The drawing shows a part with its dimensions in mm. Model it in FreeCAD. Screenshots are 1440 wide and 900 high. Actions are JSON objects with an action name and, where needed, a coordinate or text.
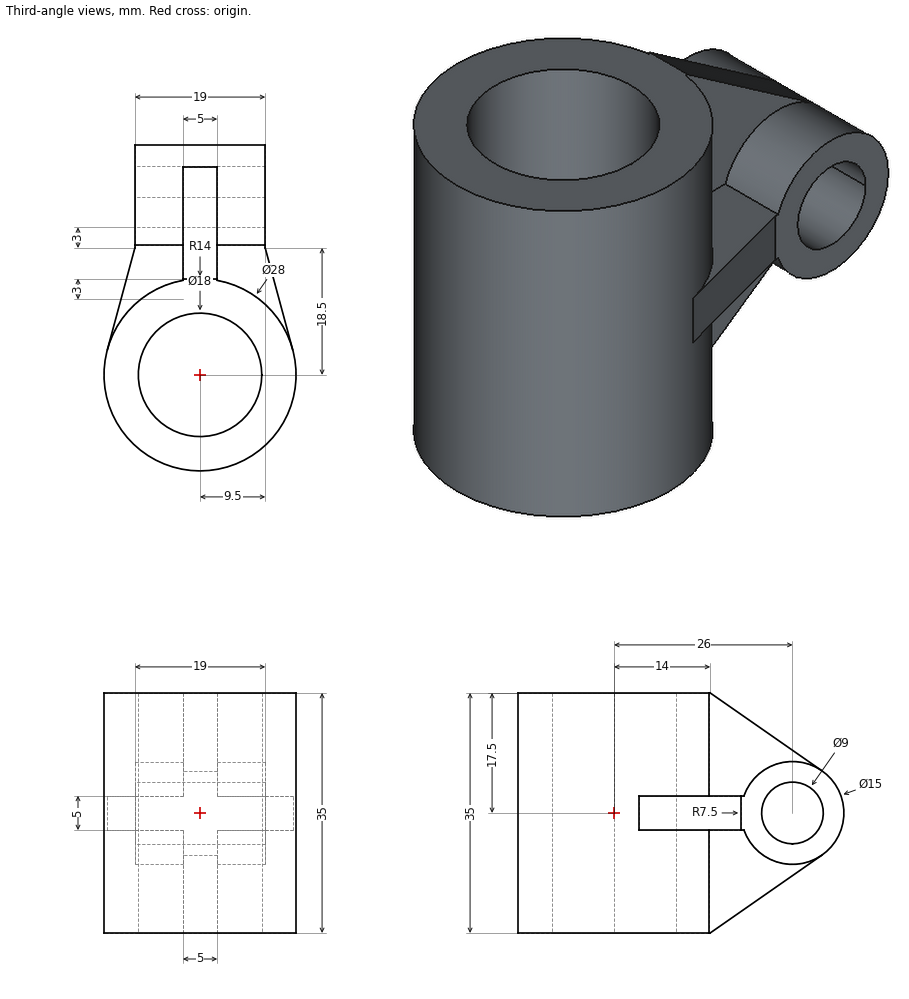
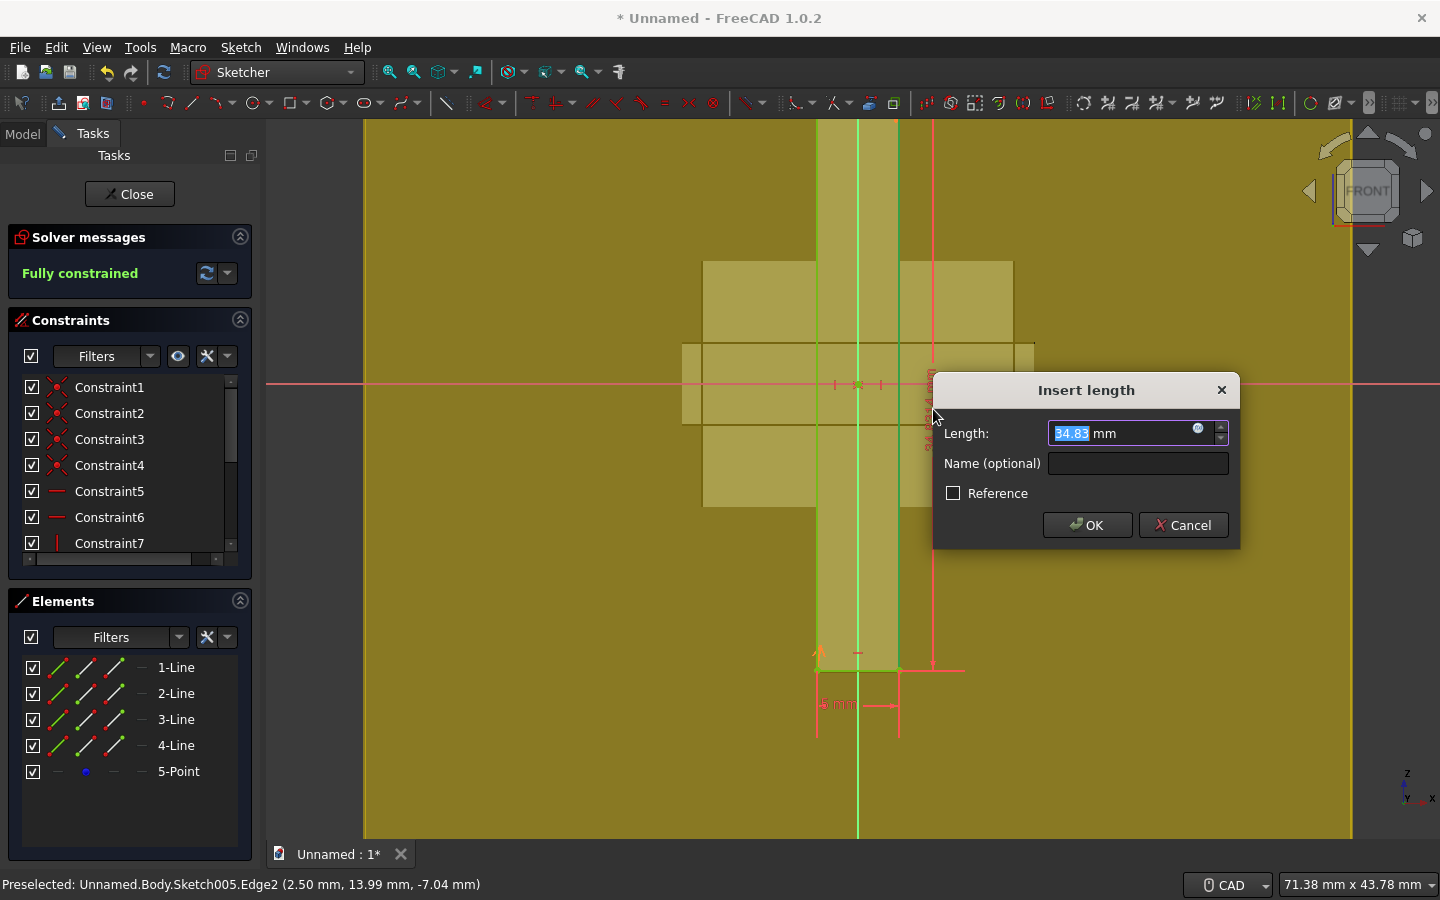
{"action": "type", "text": "35"}
{"action": "key", "text": "Return"}
{"action": "key", "text": "Escape"}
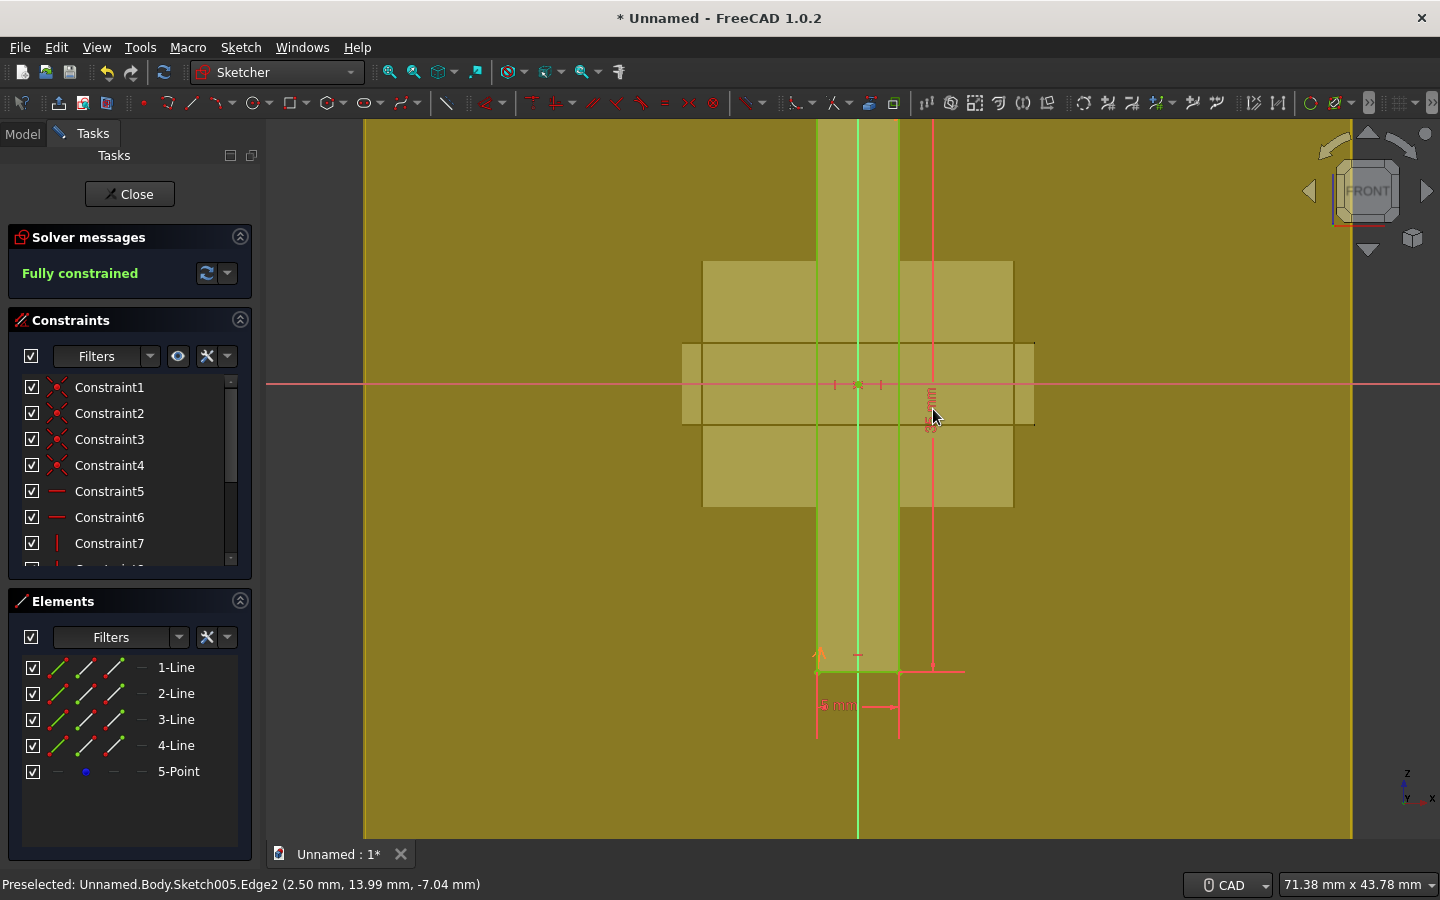
{"action": "left_click", "coordinate": [130, 194]}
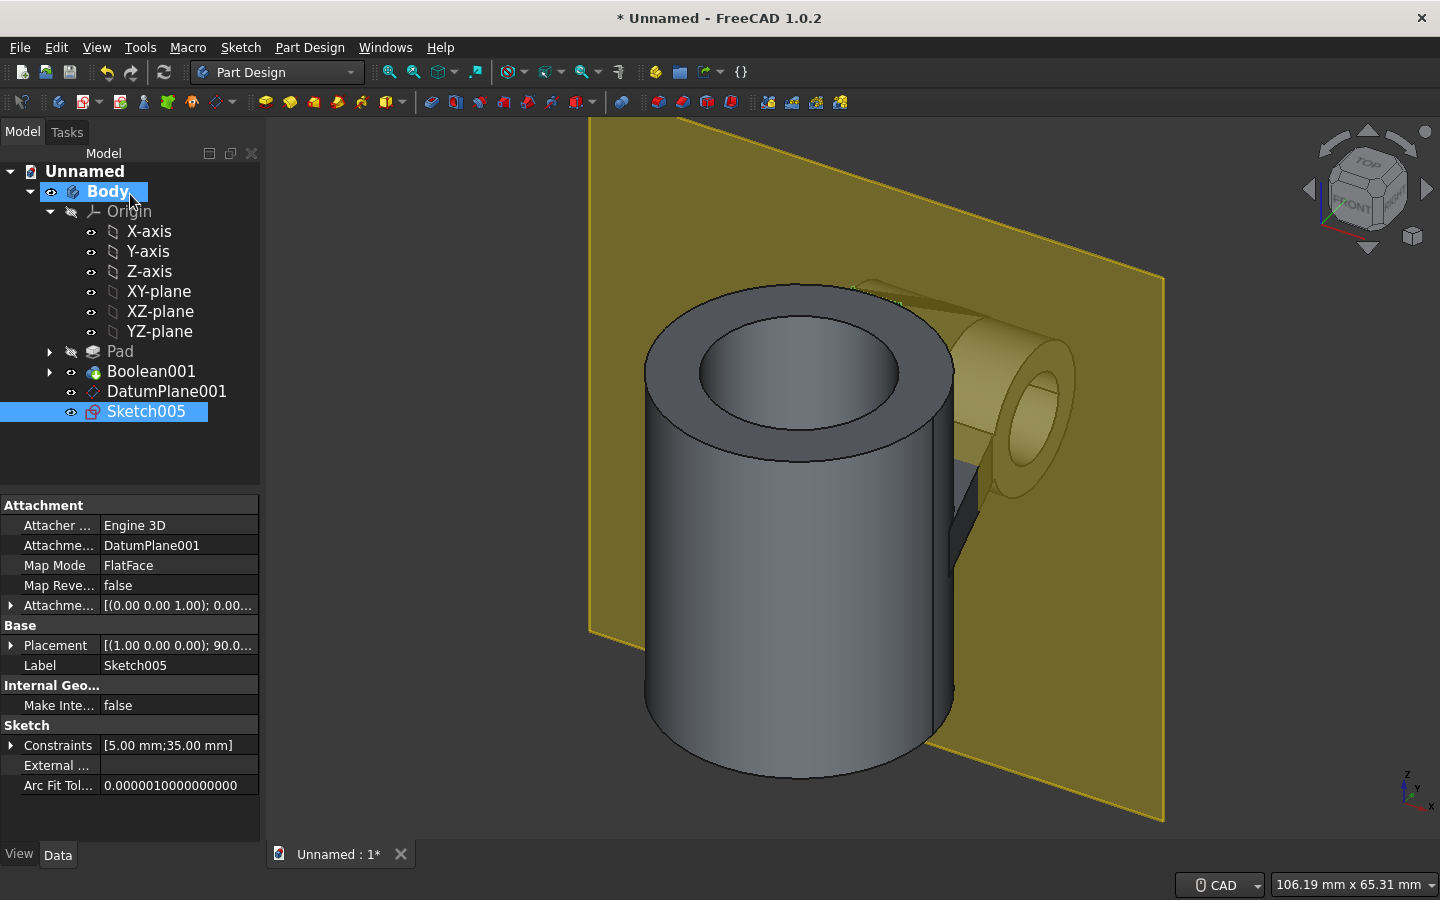
{"action": "left_click", "coordinate": [266, 102]}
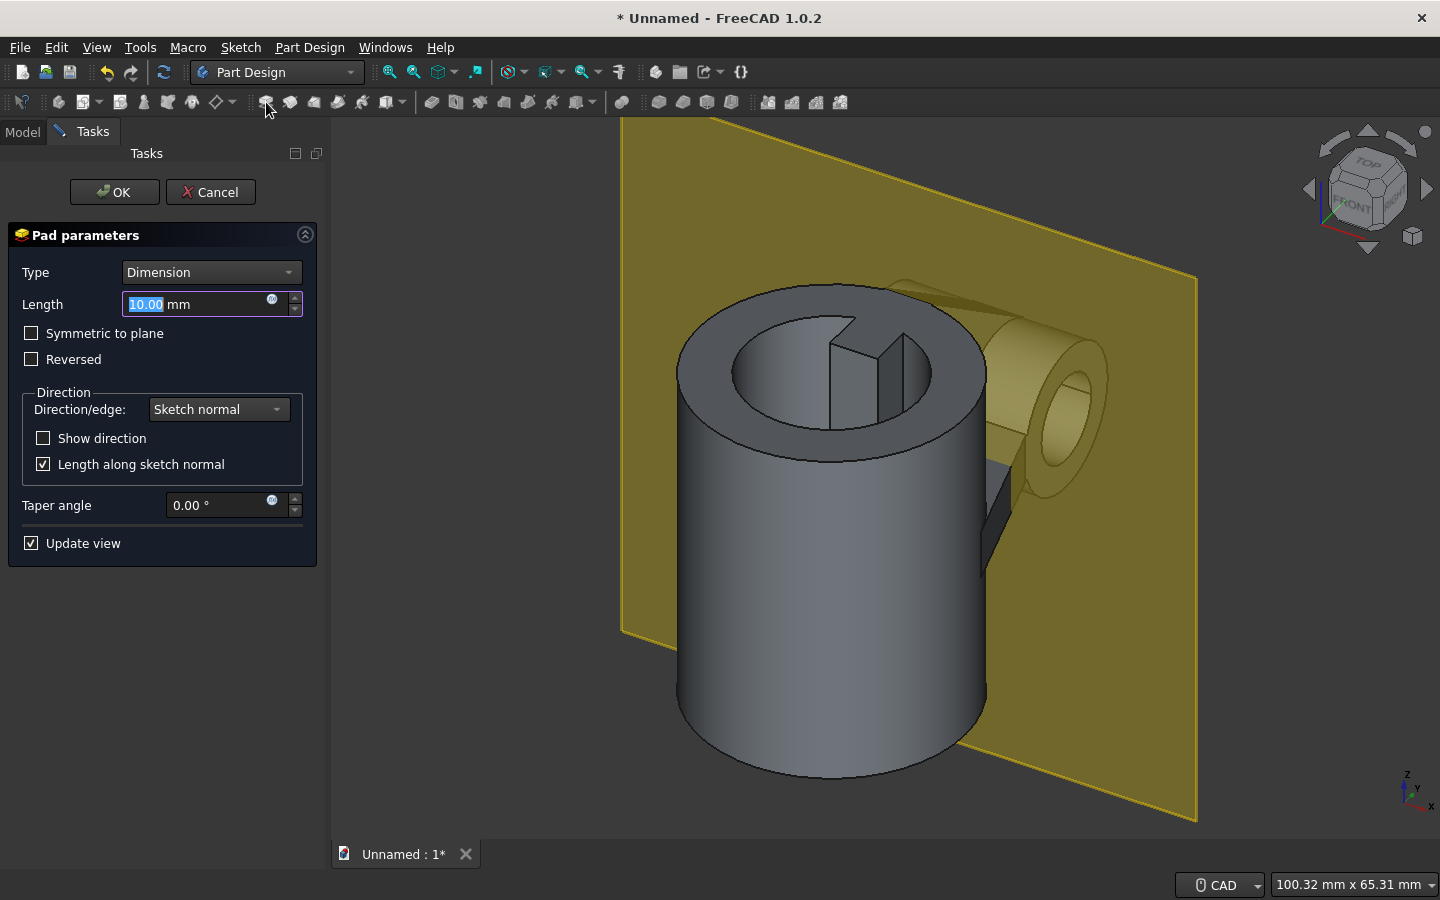
{"action": "type", "text": "3"}
{"action": "key", "text": "Tab"}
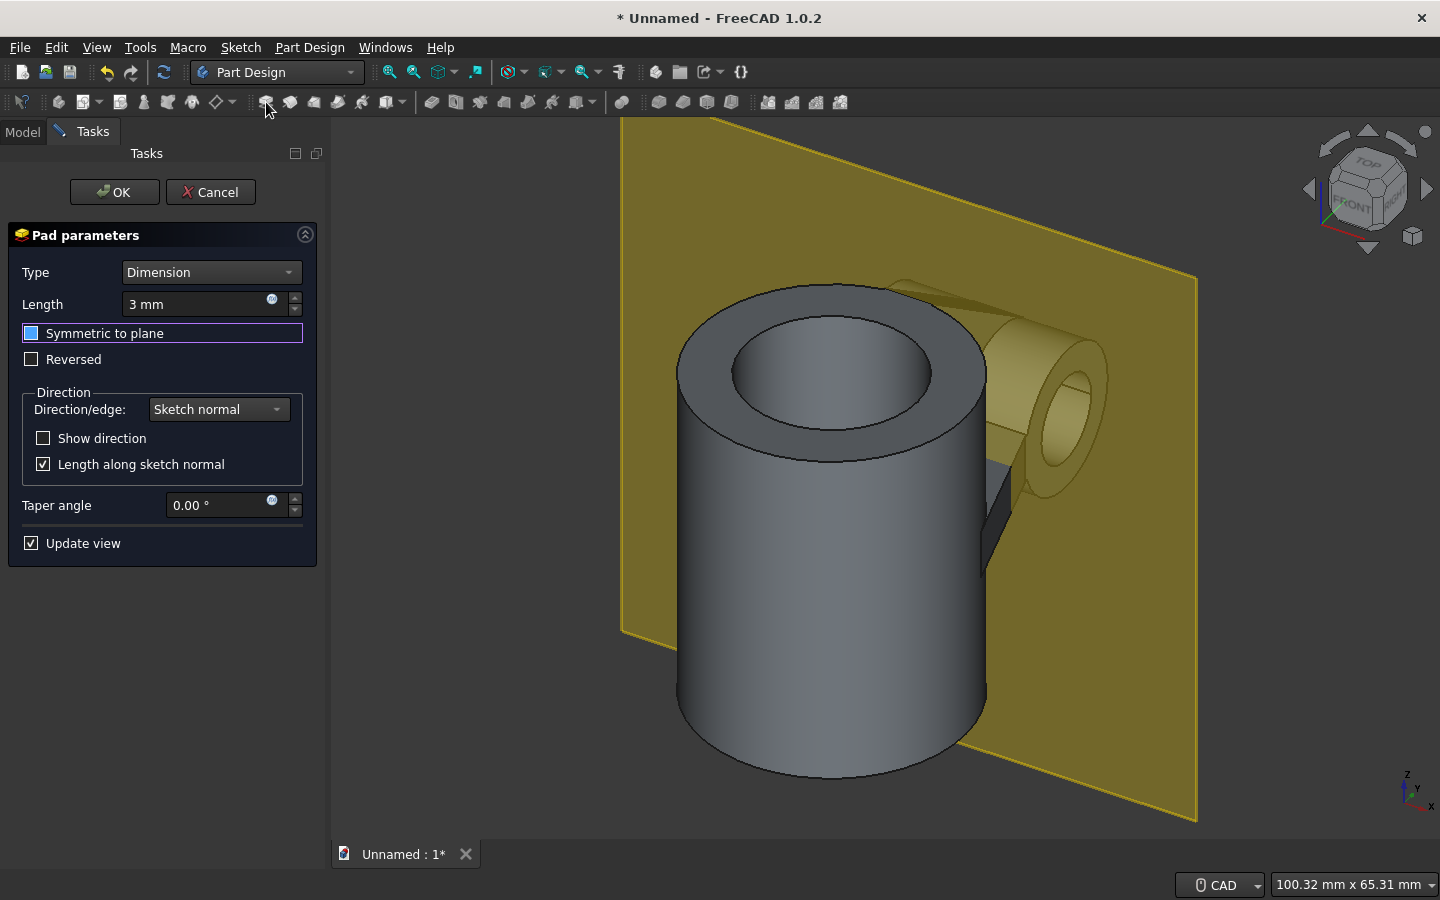
{"action": "left_click", "coordinate": [115, 192]}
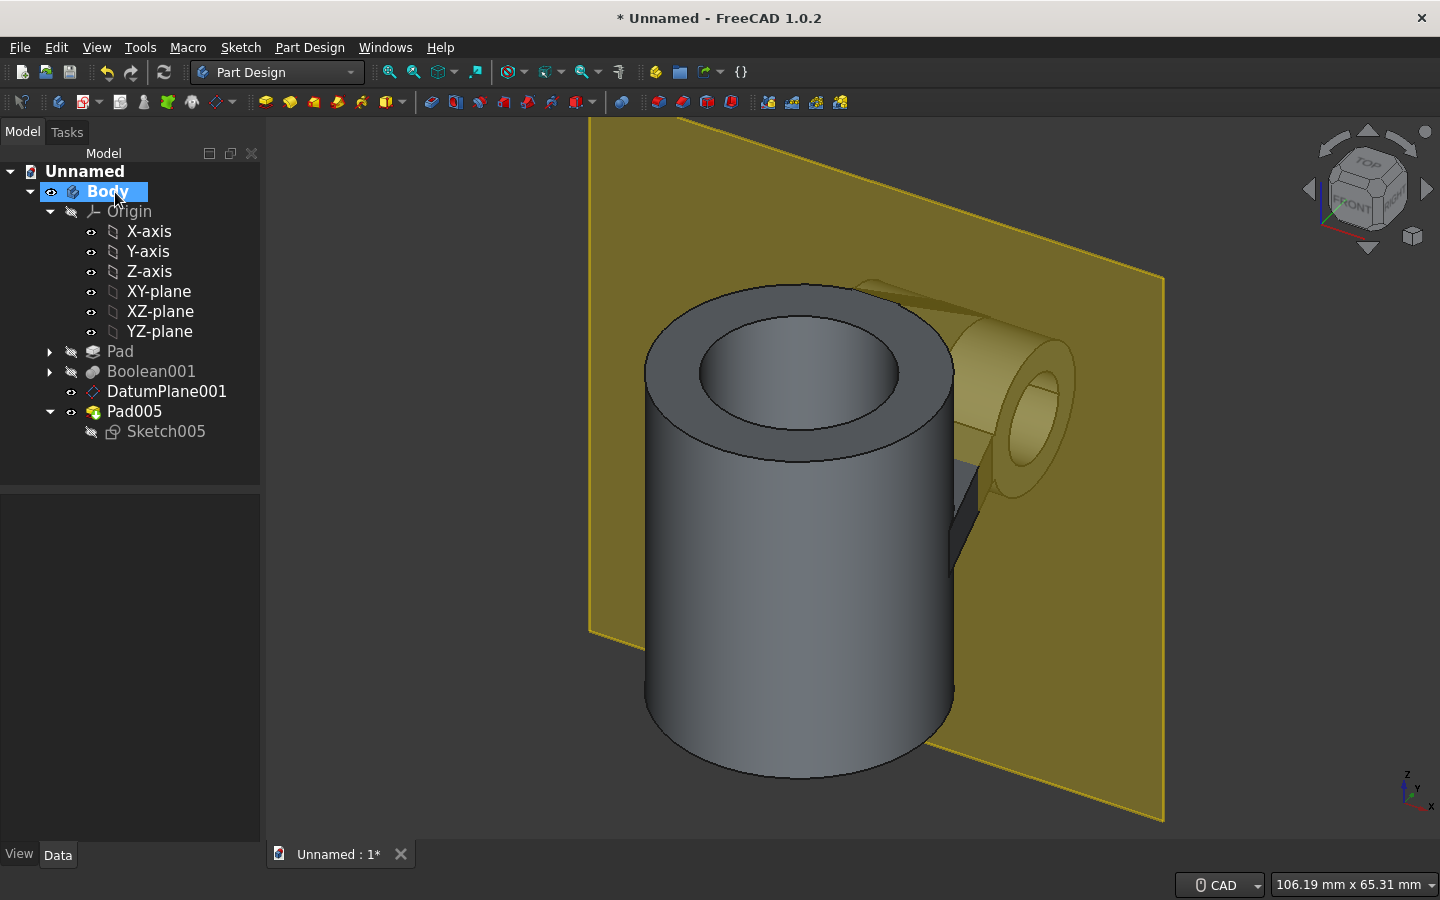
{"action": "left_click", "coordinate": [116, 392]}
{"action": "key", "text": "space"}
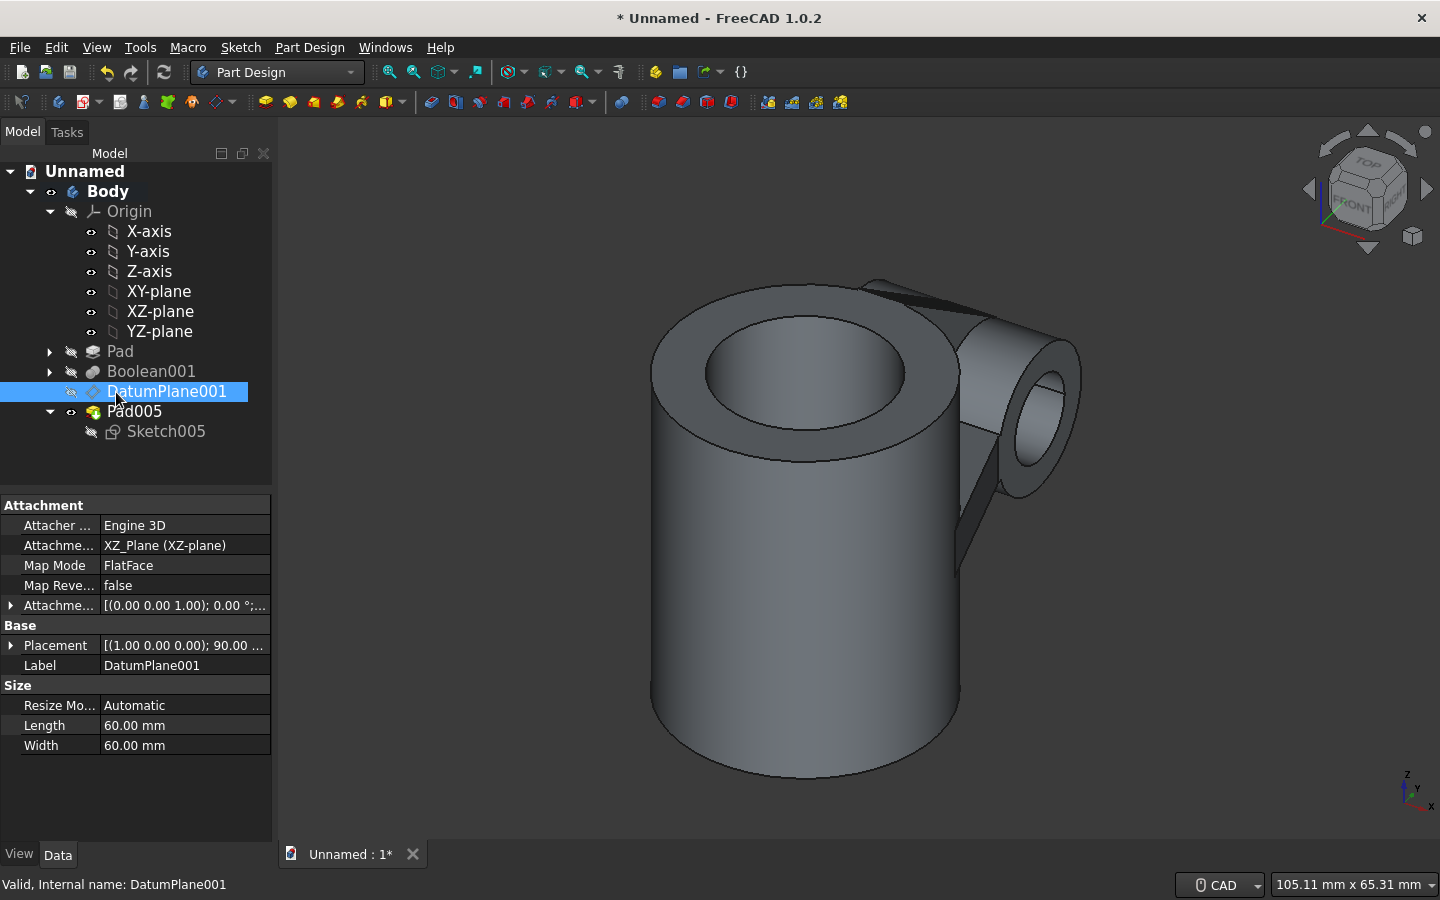
{"action": "key", "text": "0"}